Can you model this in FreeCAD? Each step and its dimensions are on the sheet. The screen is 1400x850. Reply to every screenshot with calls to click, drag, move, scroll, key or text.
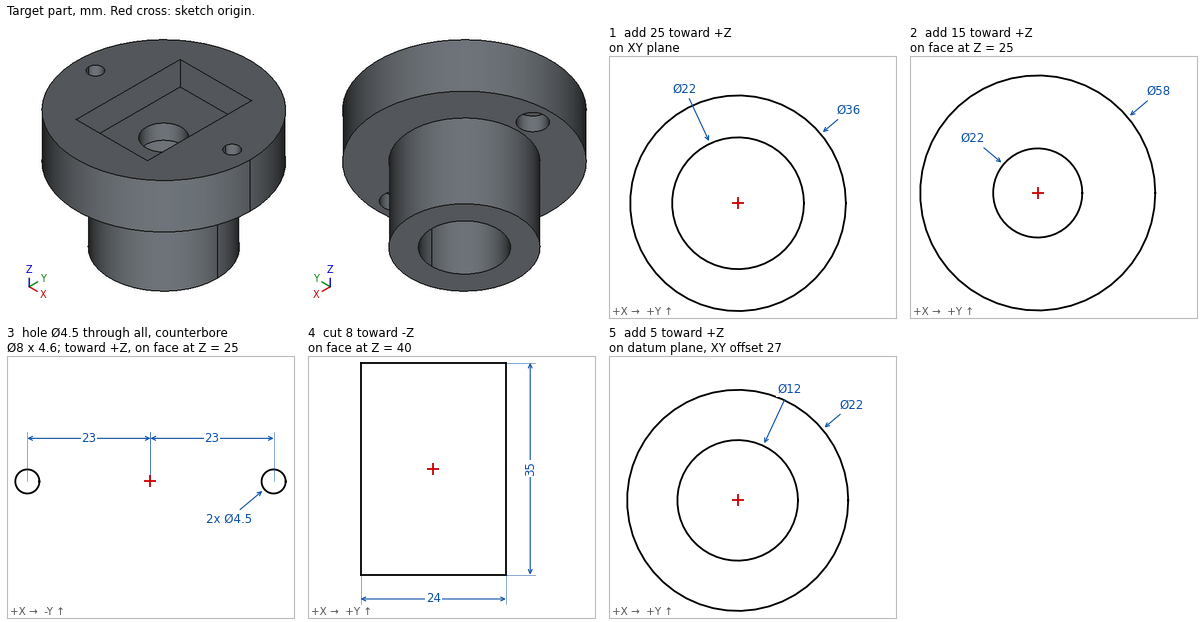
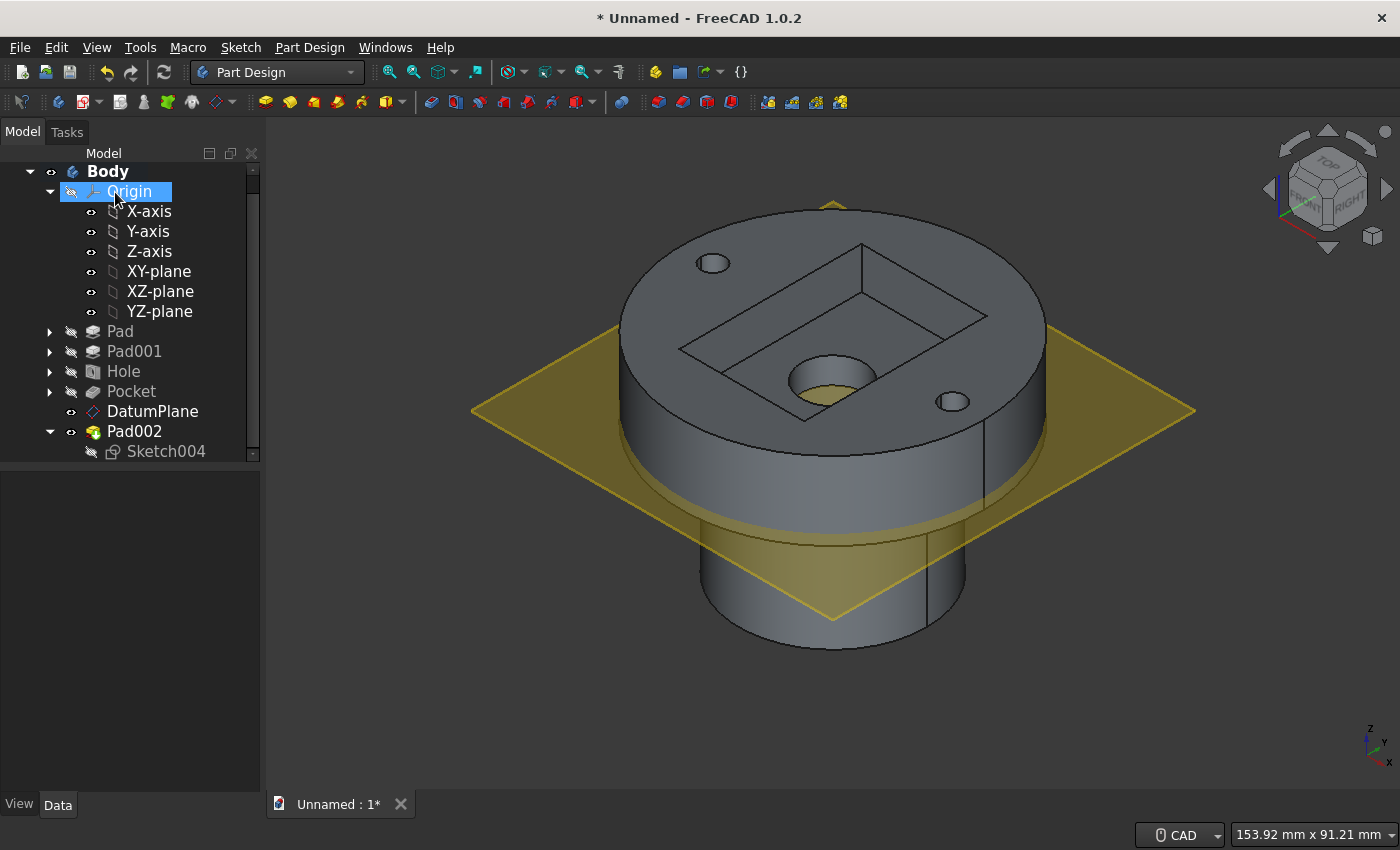
click(116, 412)
key(space)